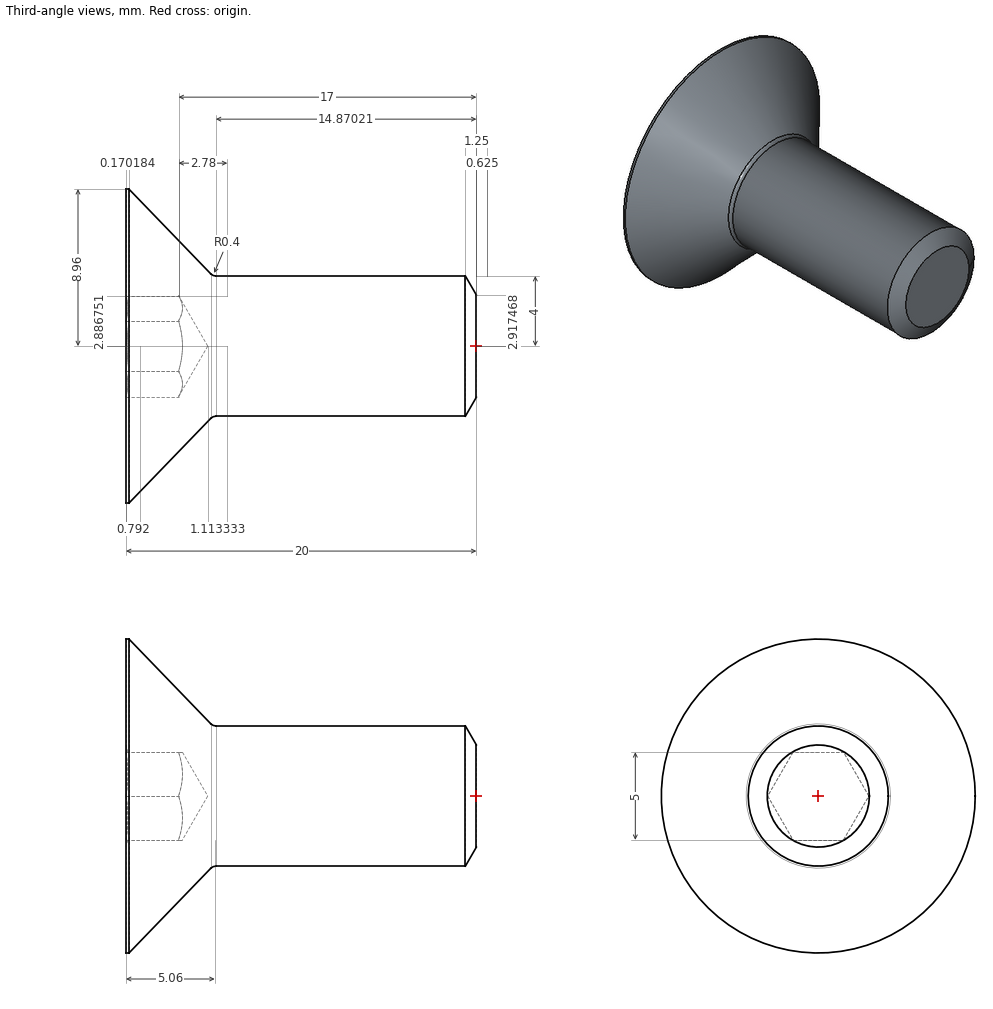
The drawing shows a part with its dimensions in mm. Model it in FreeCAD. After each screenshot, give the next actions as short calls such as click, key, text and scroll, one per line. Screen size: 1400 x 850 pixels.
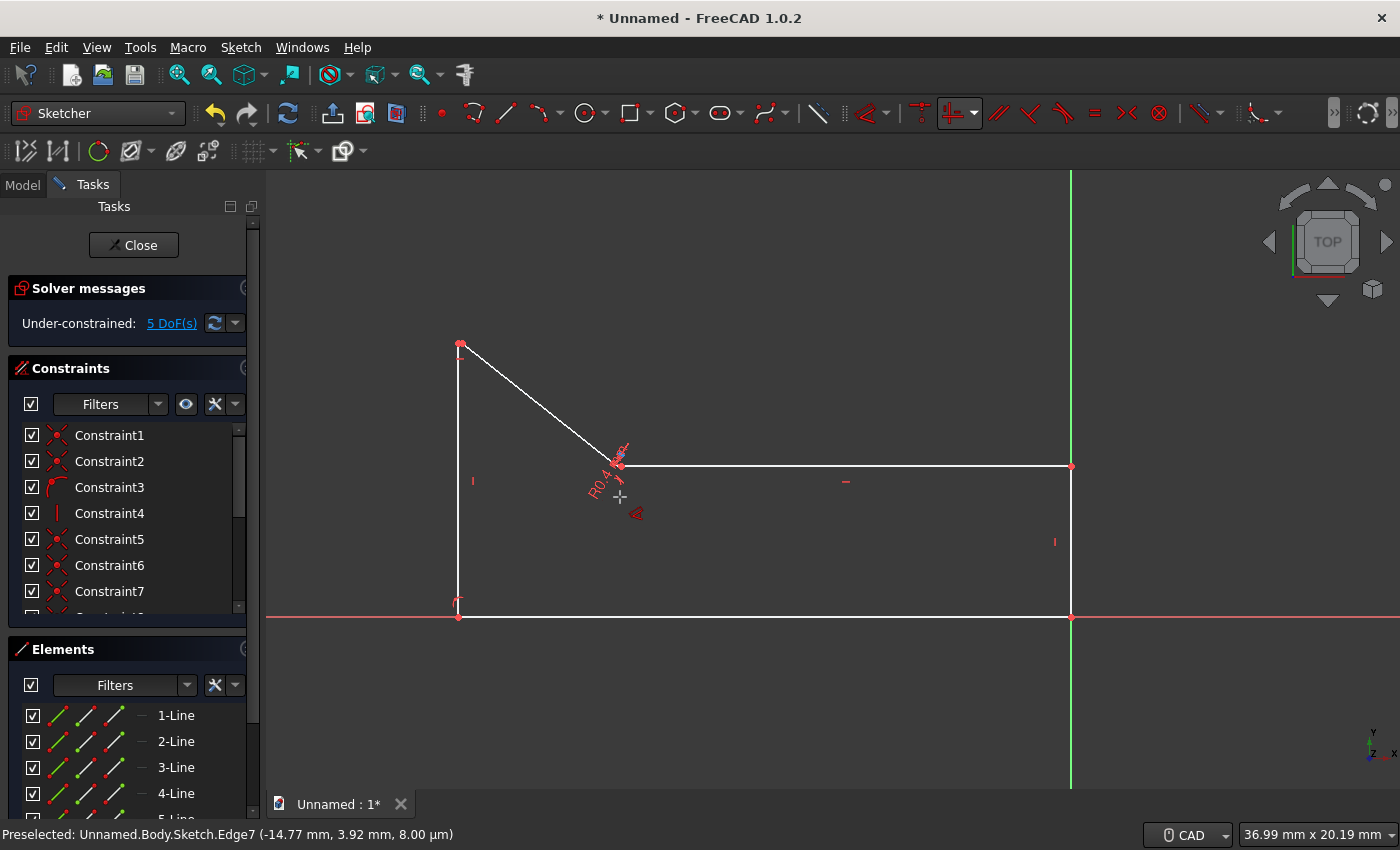
click(1071, 572)
click(1105, 542)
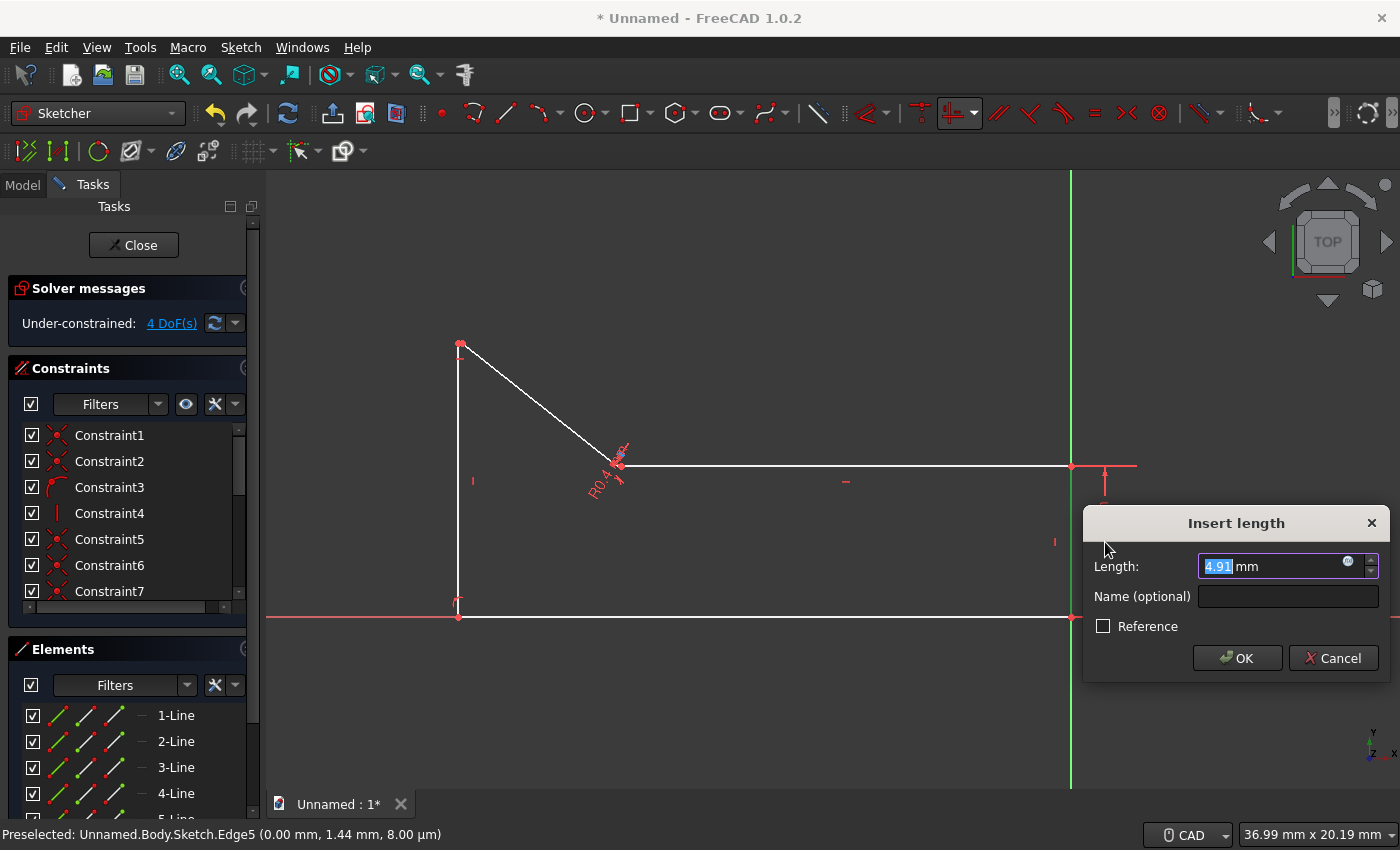
text(4)
key(Return)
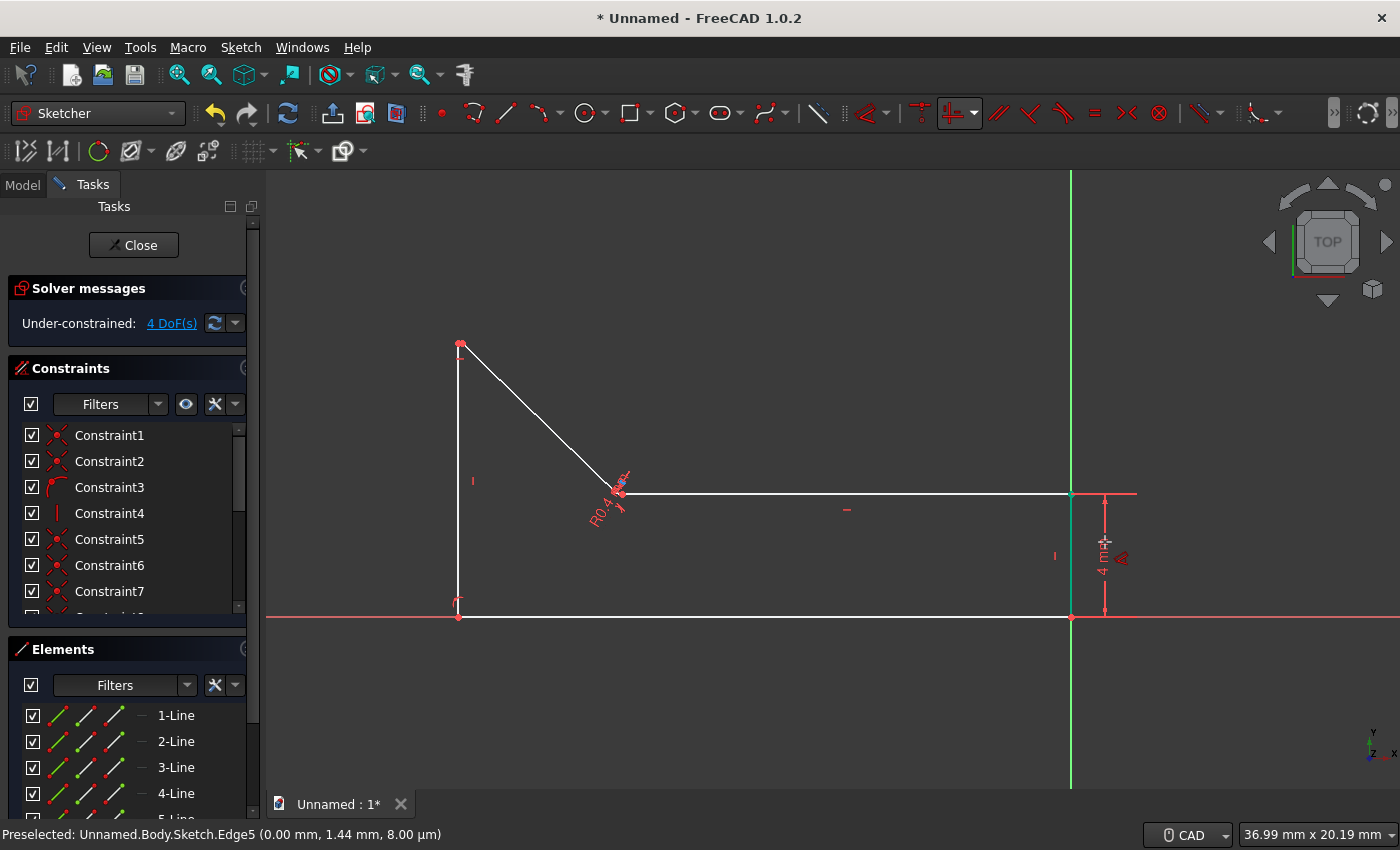
click(642, 617)
click(765, 651)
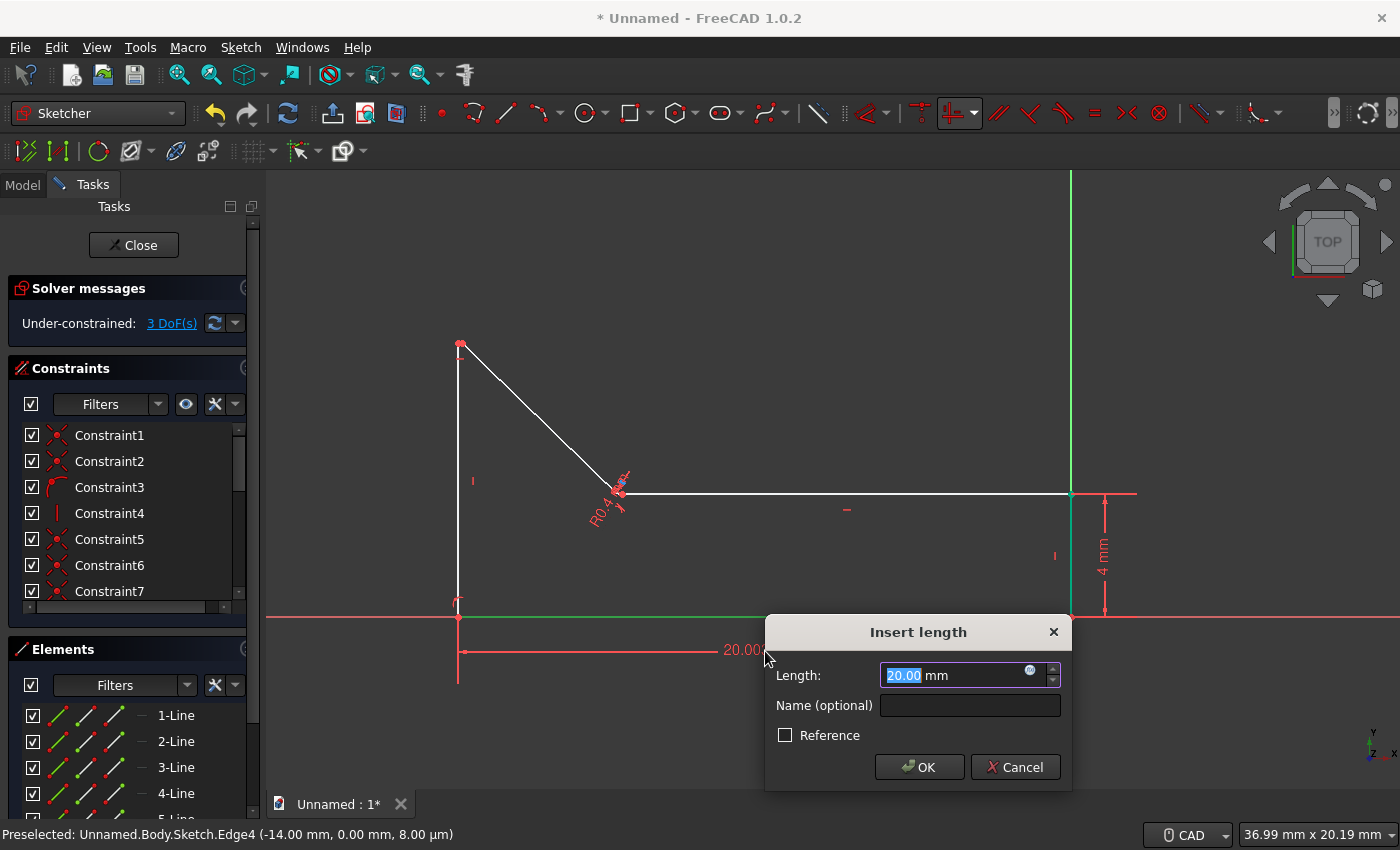
text(20)
key(Return)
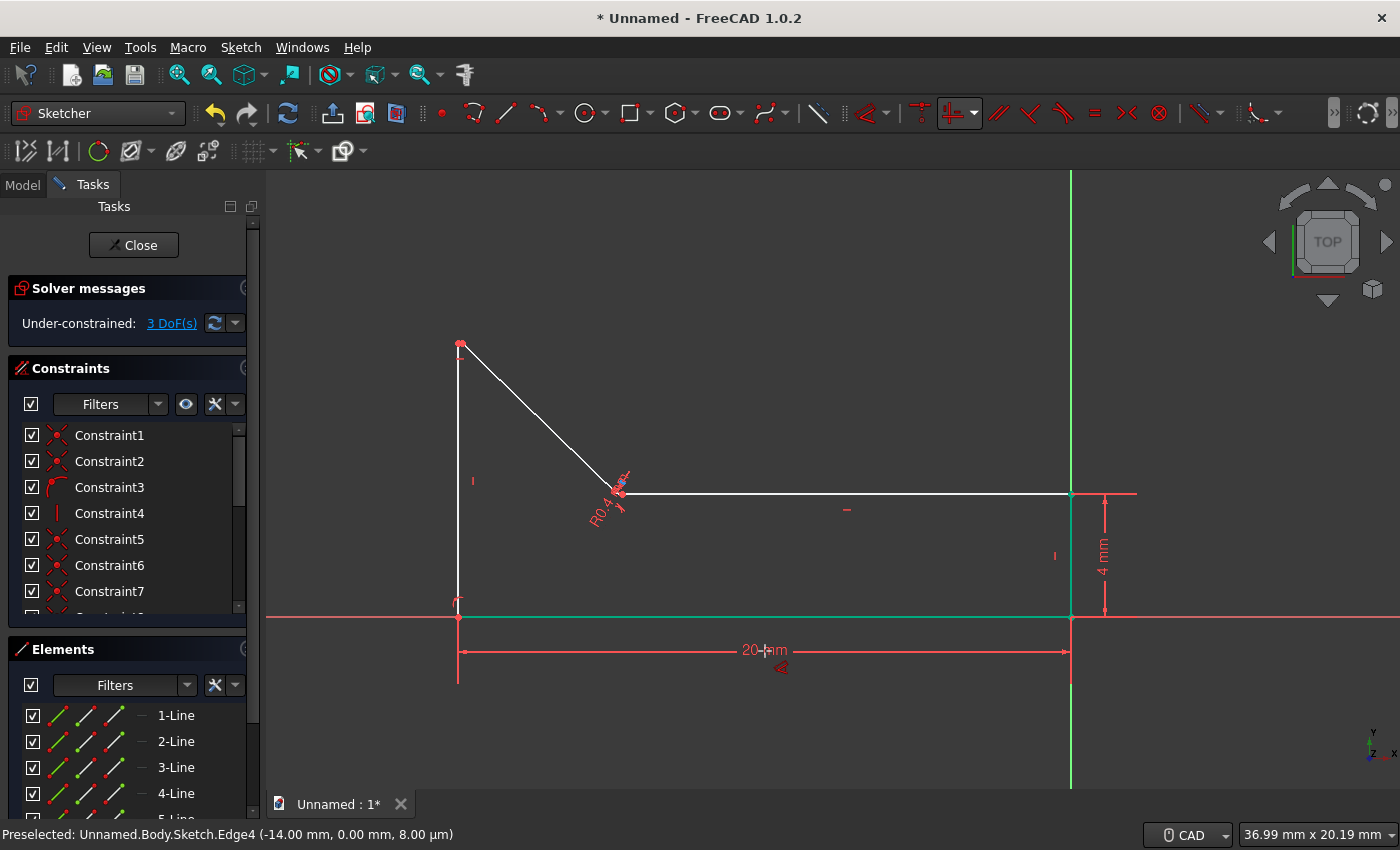
click(458, 426)
click(424, 480)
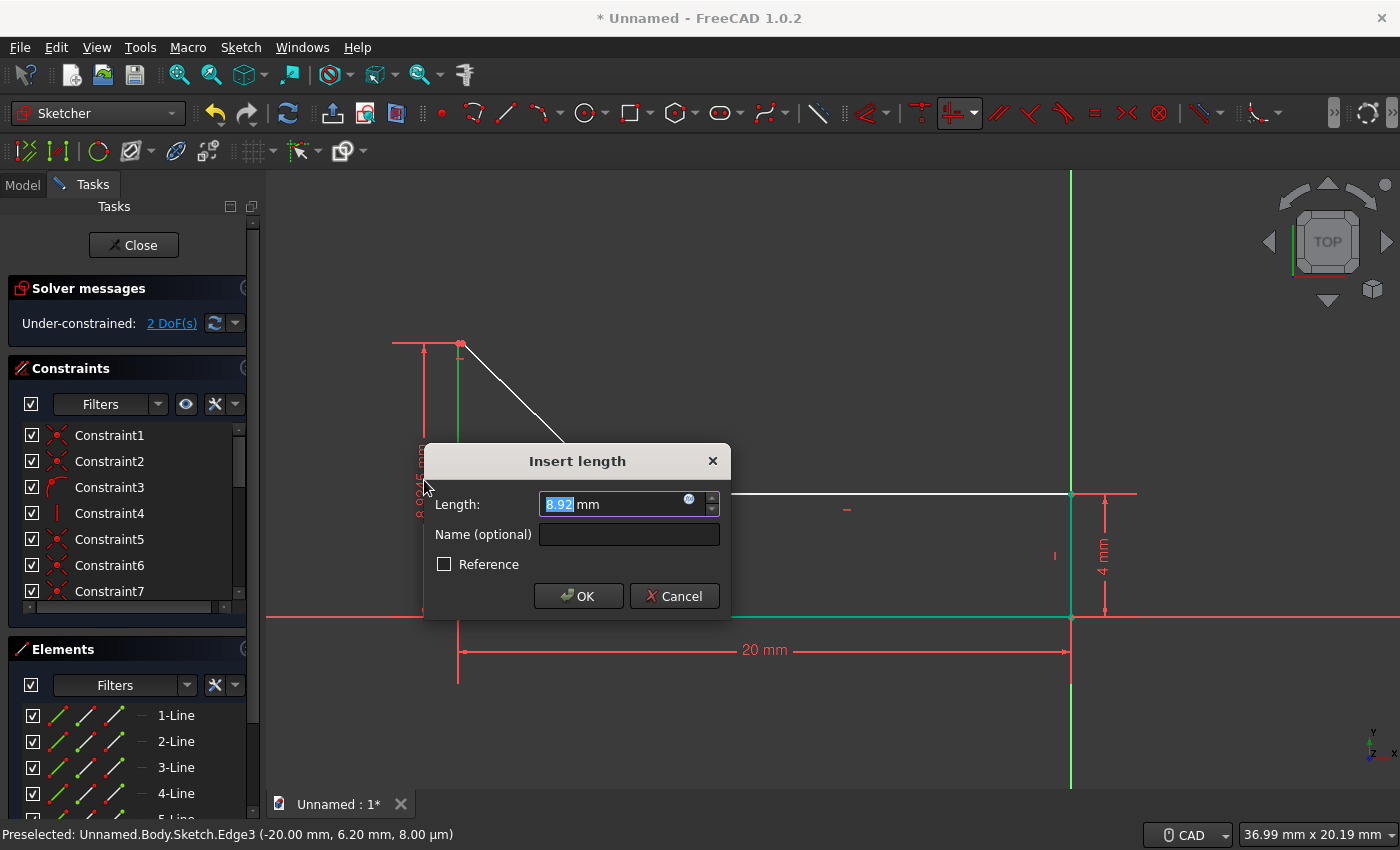
text(8.96)
key(Return)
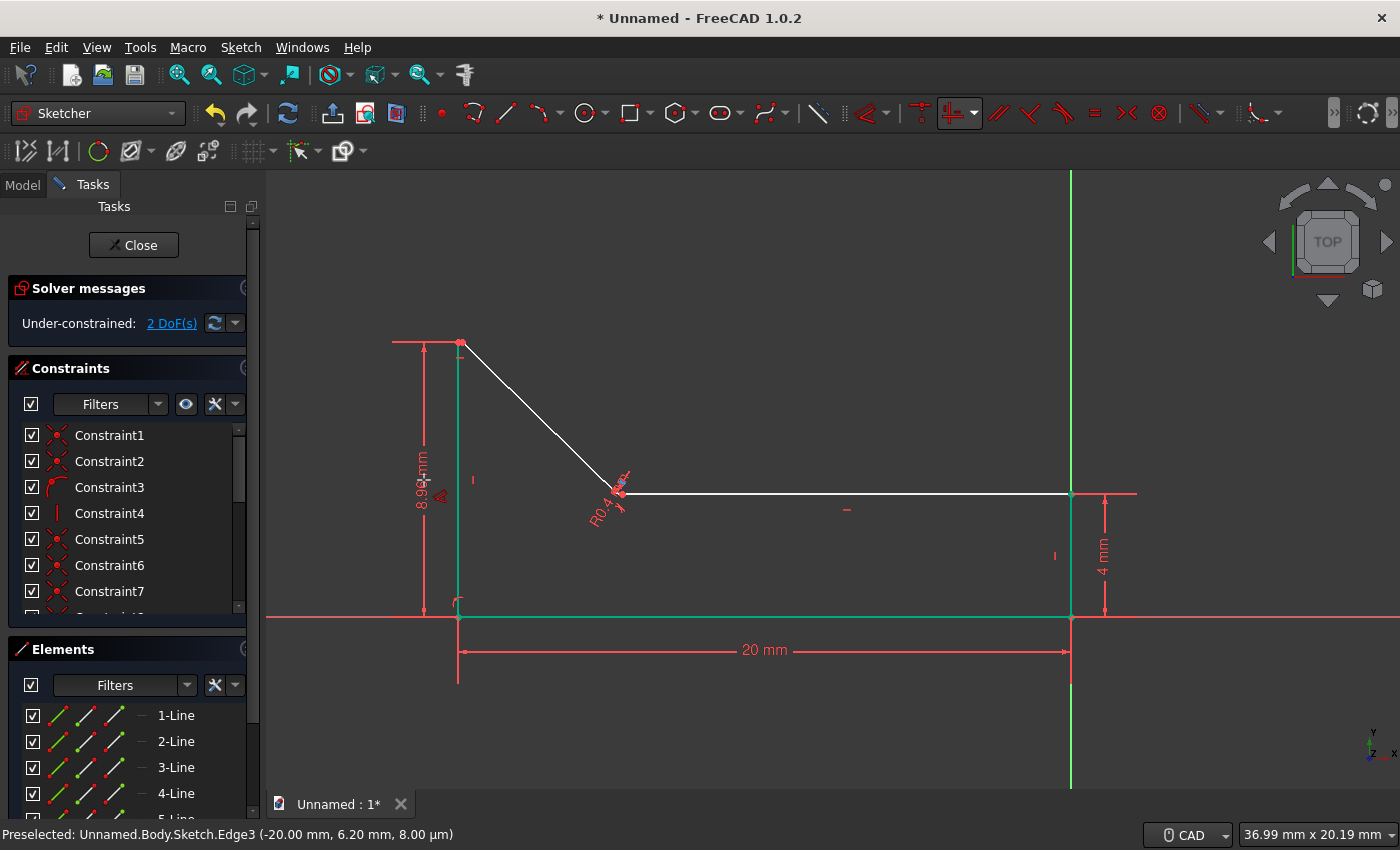
scroll(460, 342, up, 11)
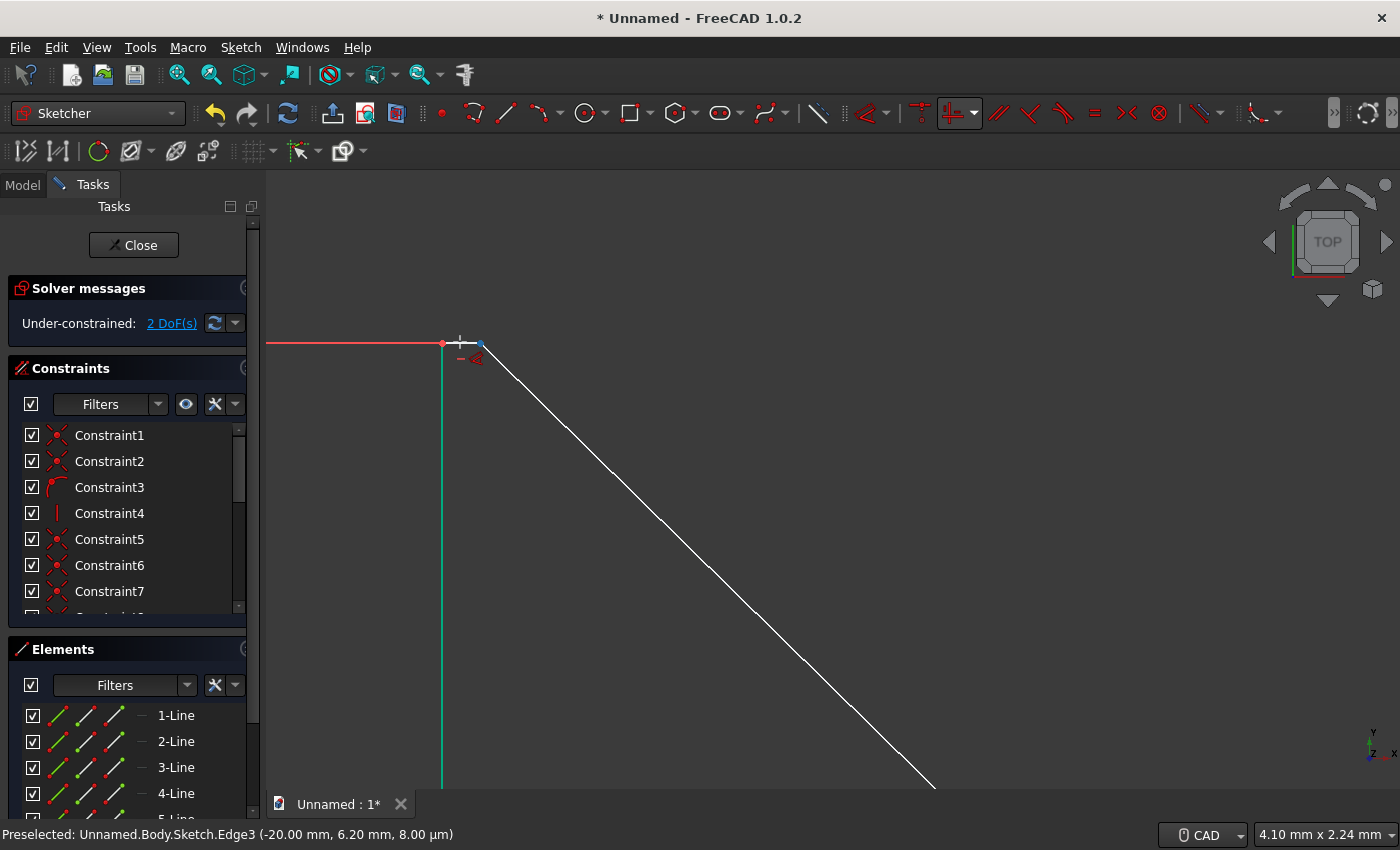
click(461, 343)
click(461, 309)